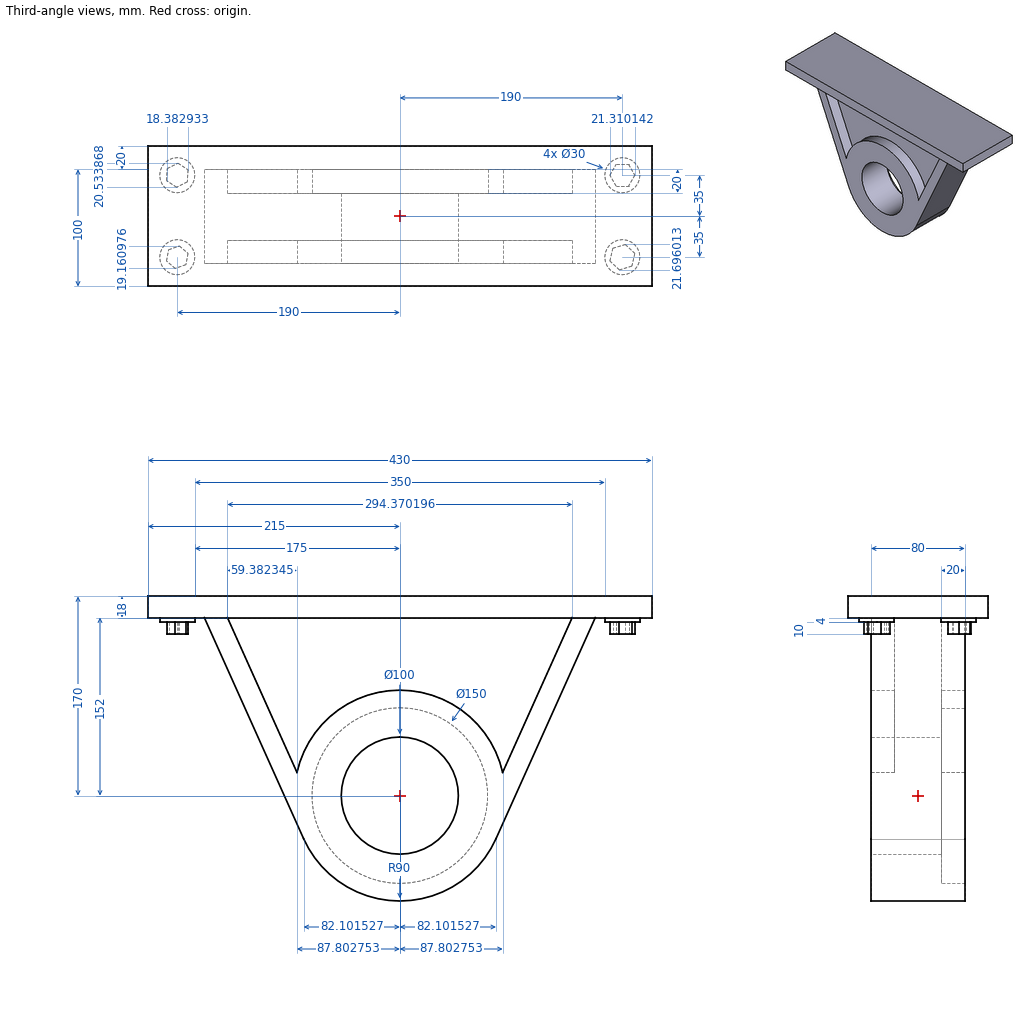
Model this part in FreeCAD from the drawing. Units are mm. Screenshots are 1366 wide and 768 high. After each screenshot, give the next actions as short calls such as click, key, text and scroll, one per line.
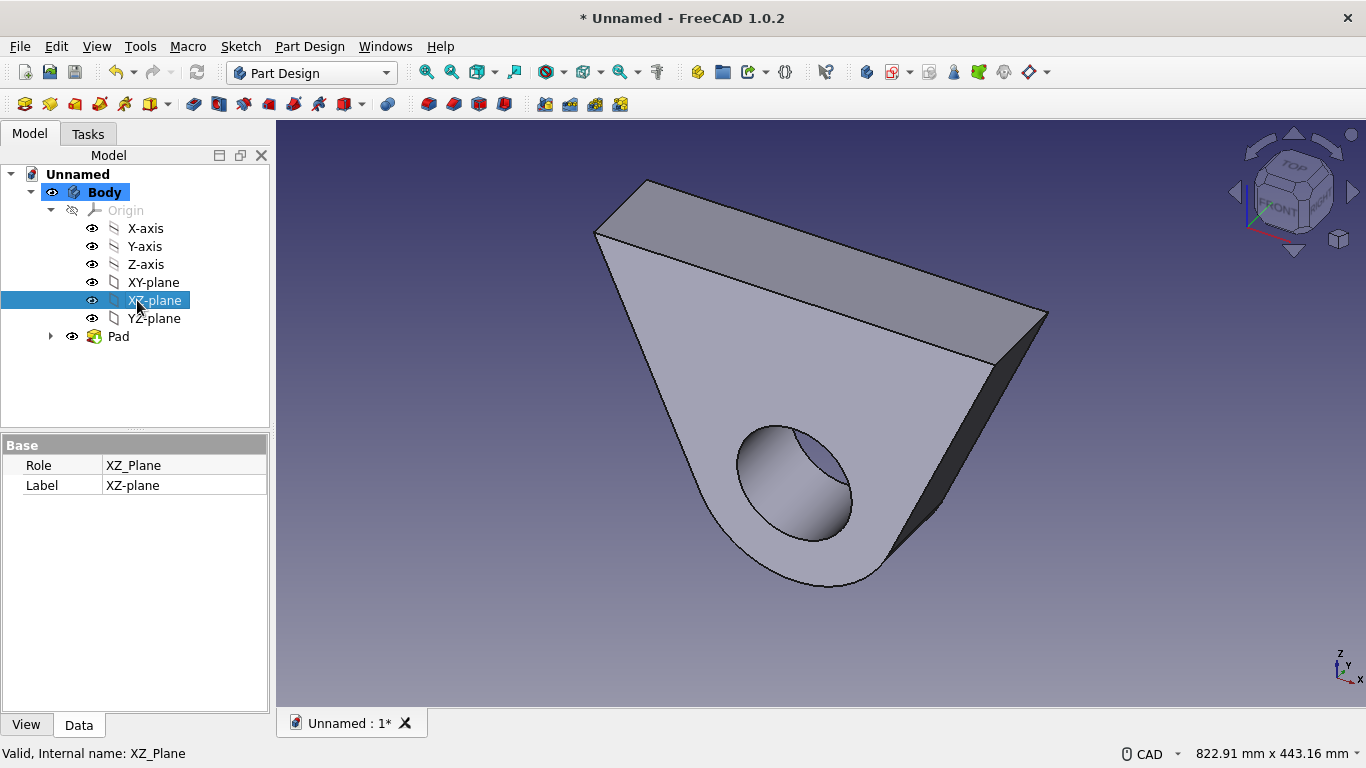
click(1028, 72)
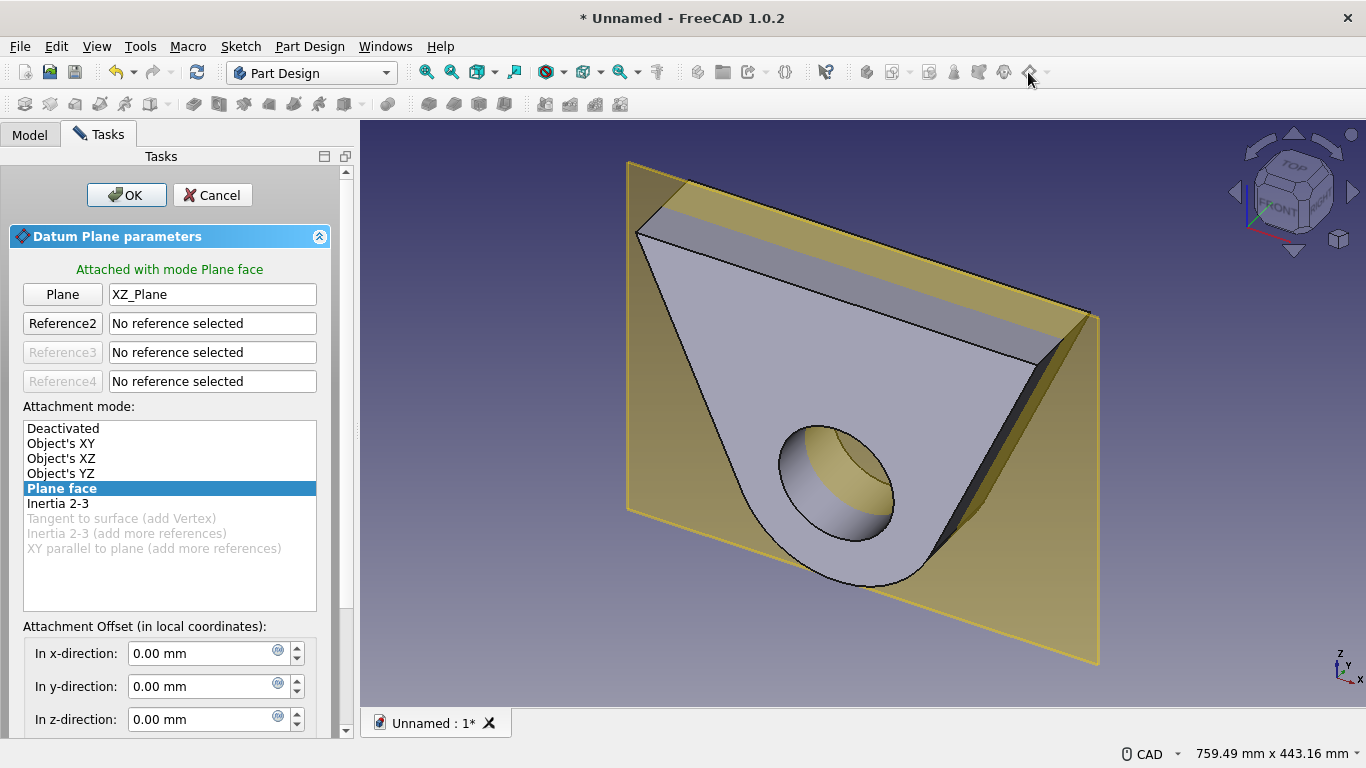
triple_click(210, 720)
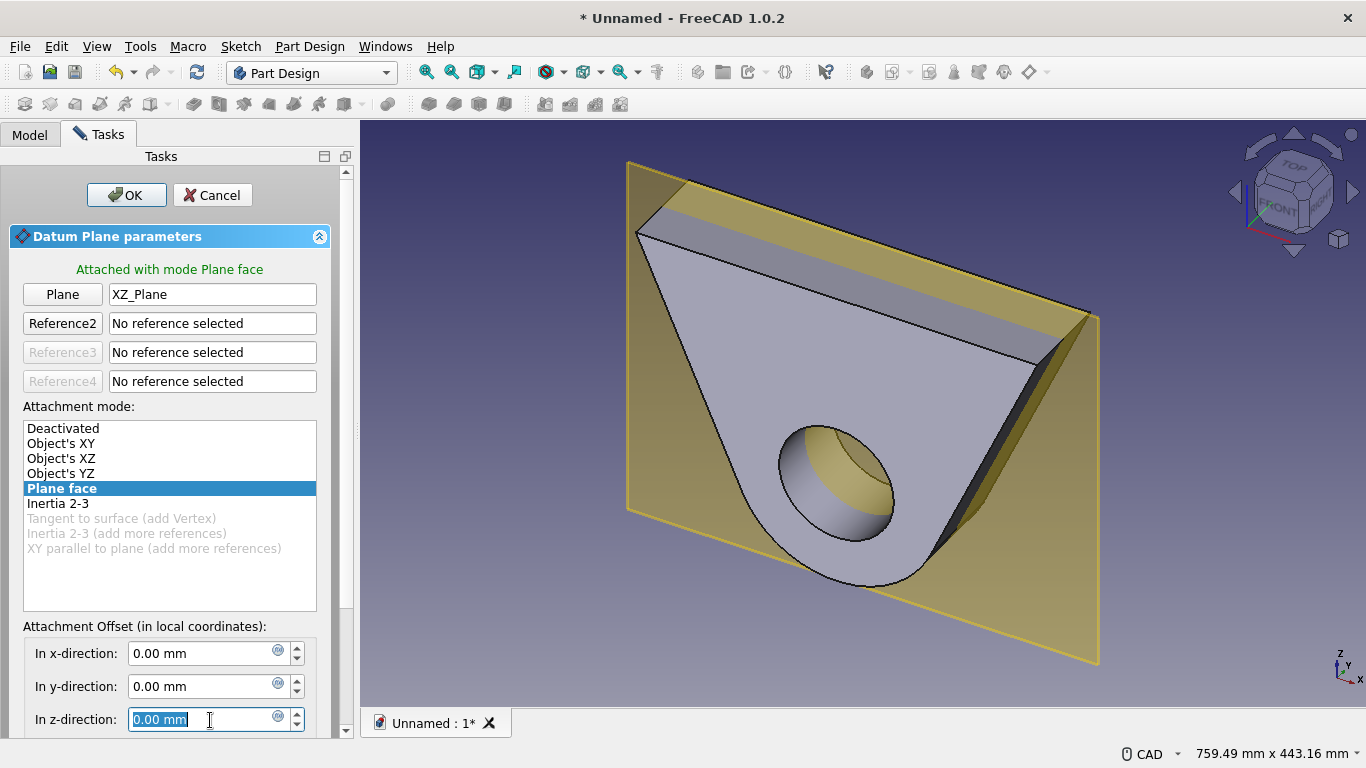
text(-20)
key(Tab)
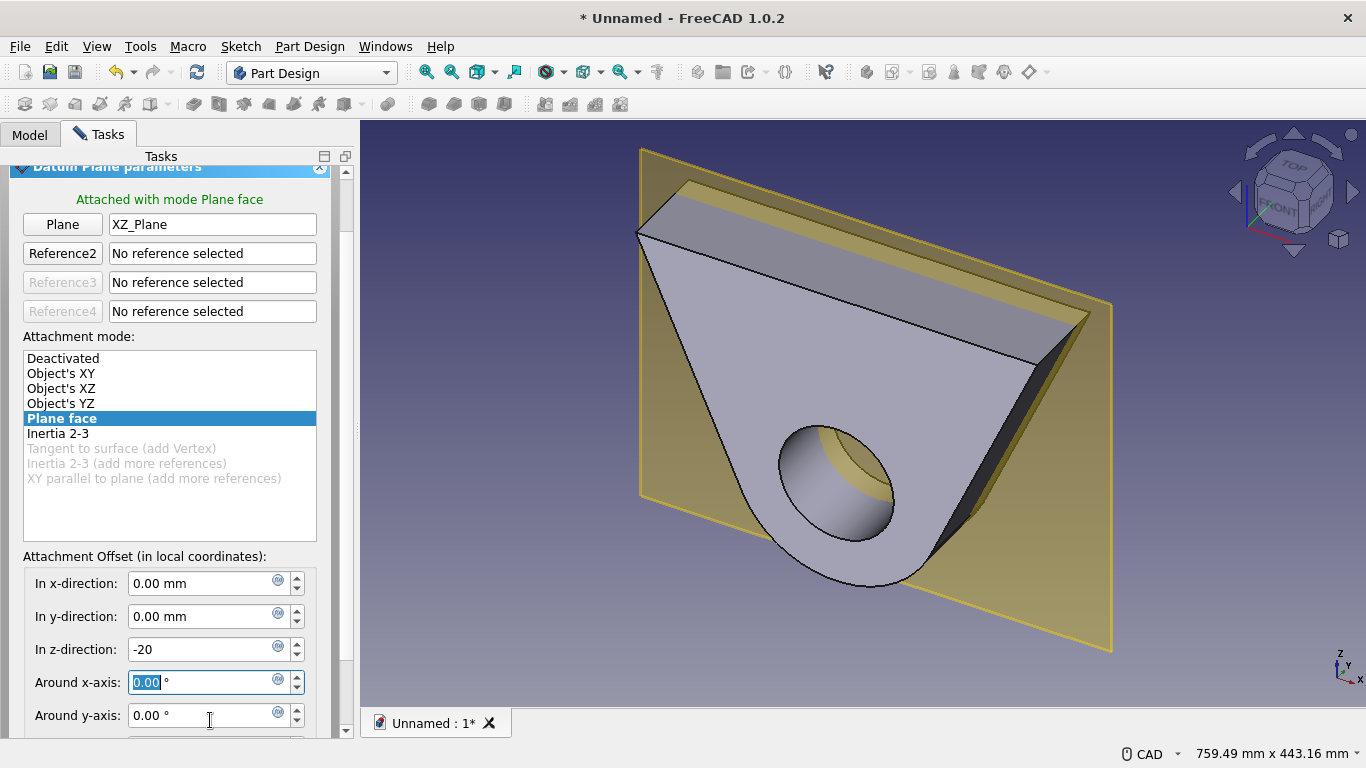
scroll(346, 452, up, 2)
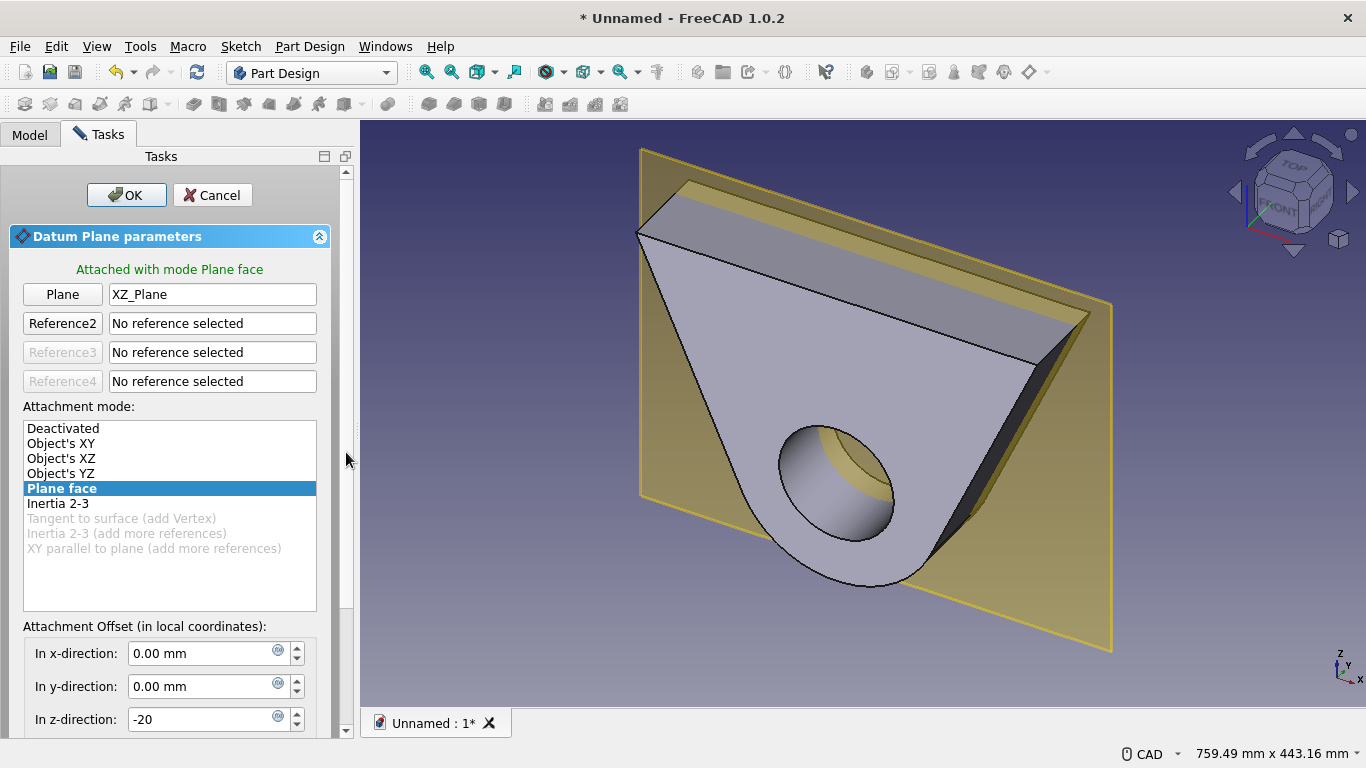
click(127, 195)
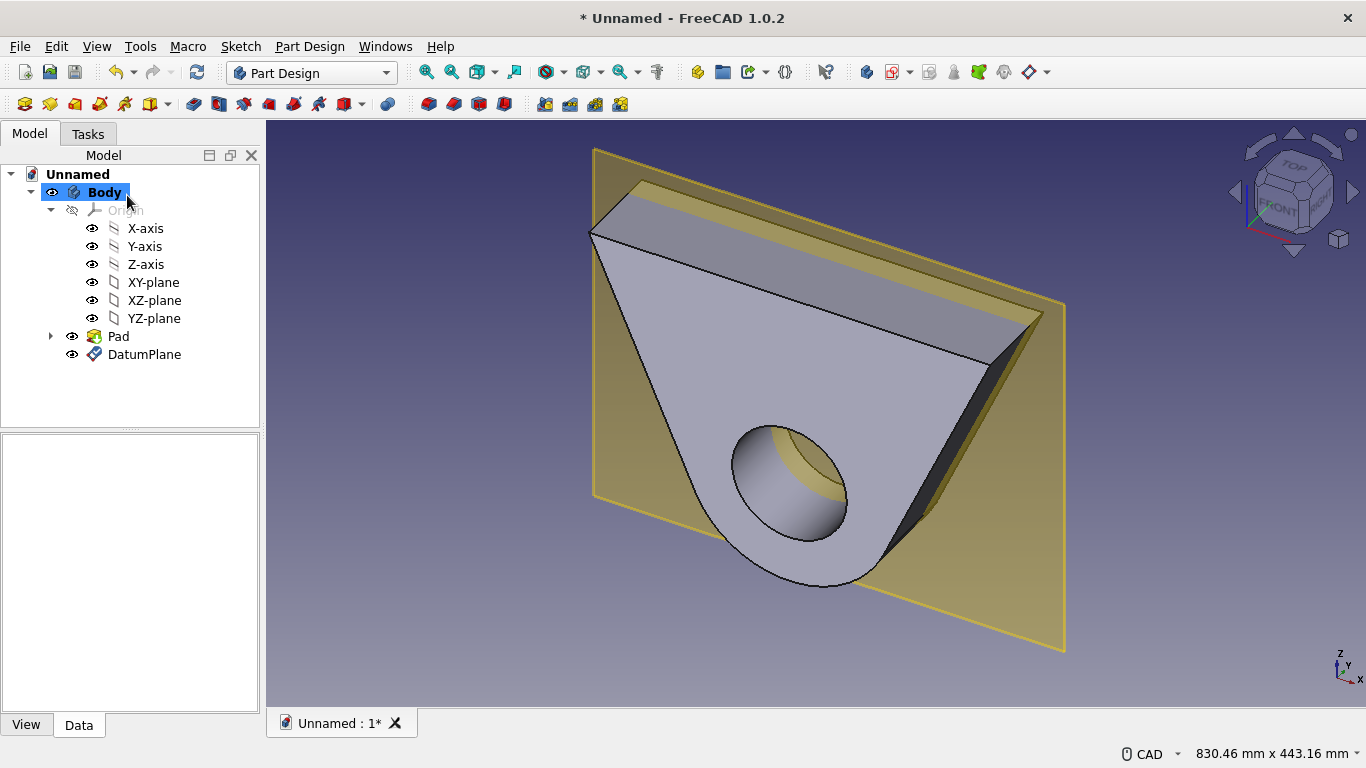
click(117, 354)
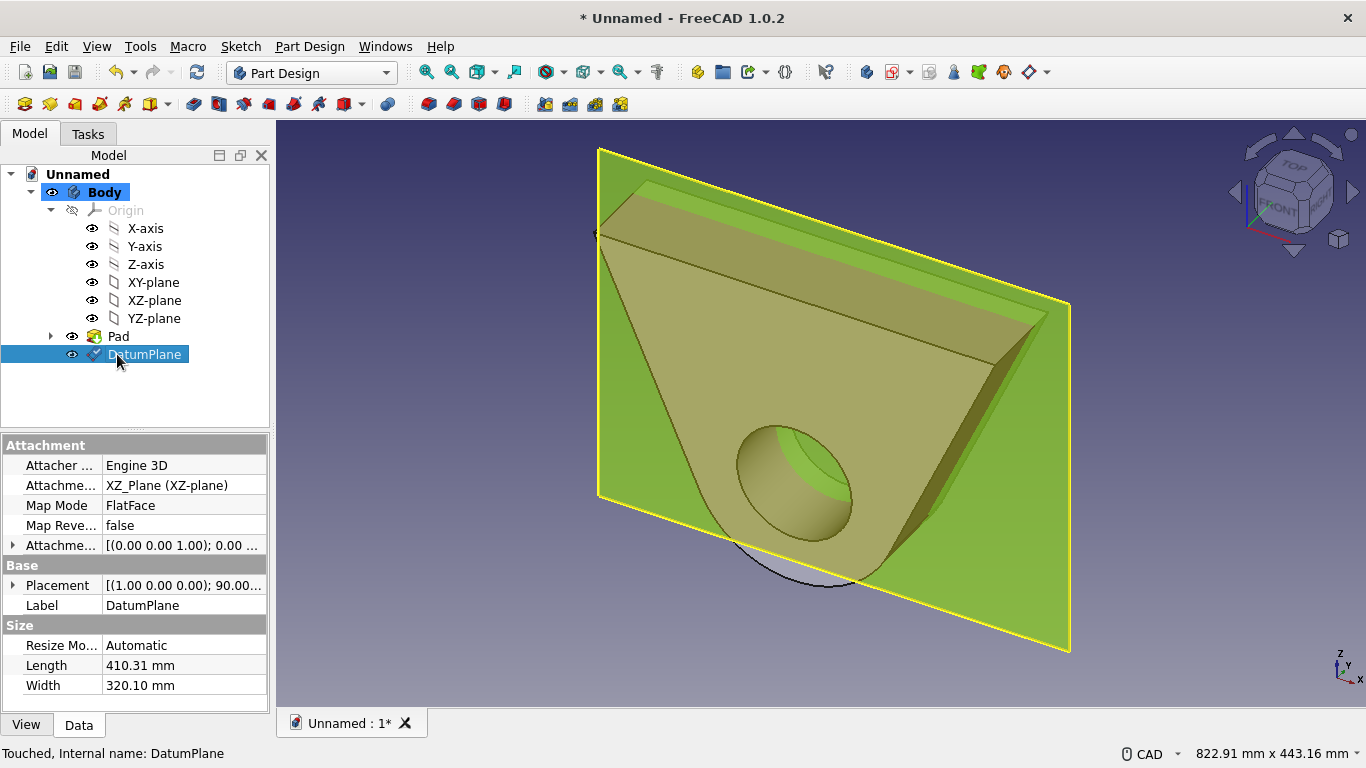
click(892, 72)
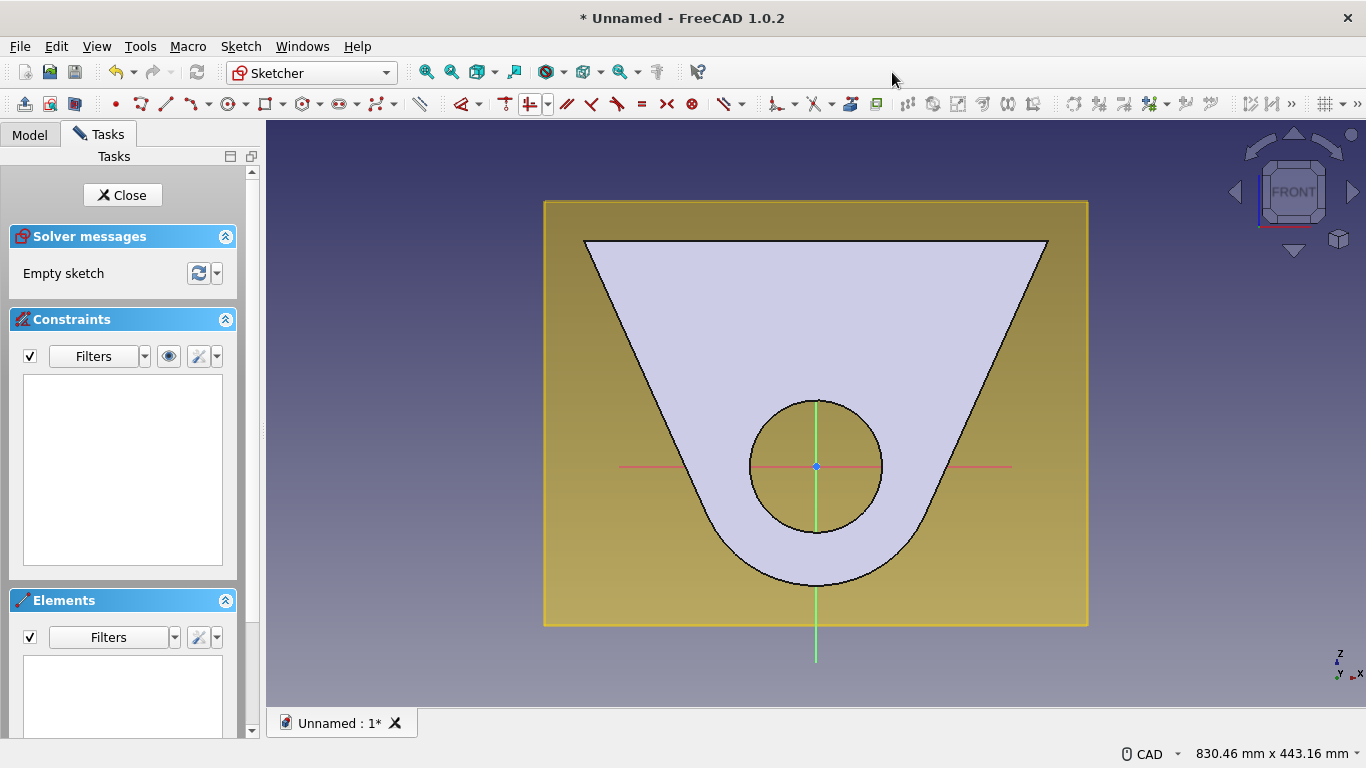
click(75, 104)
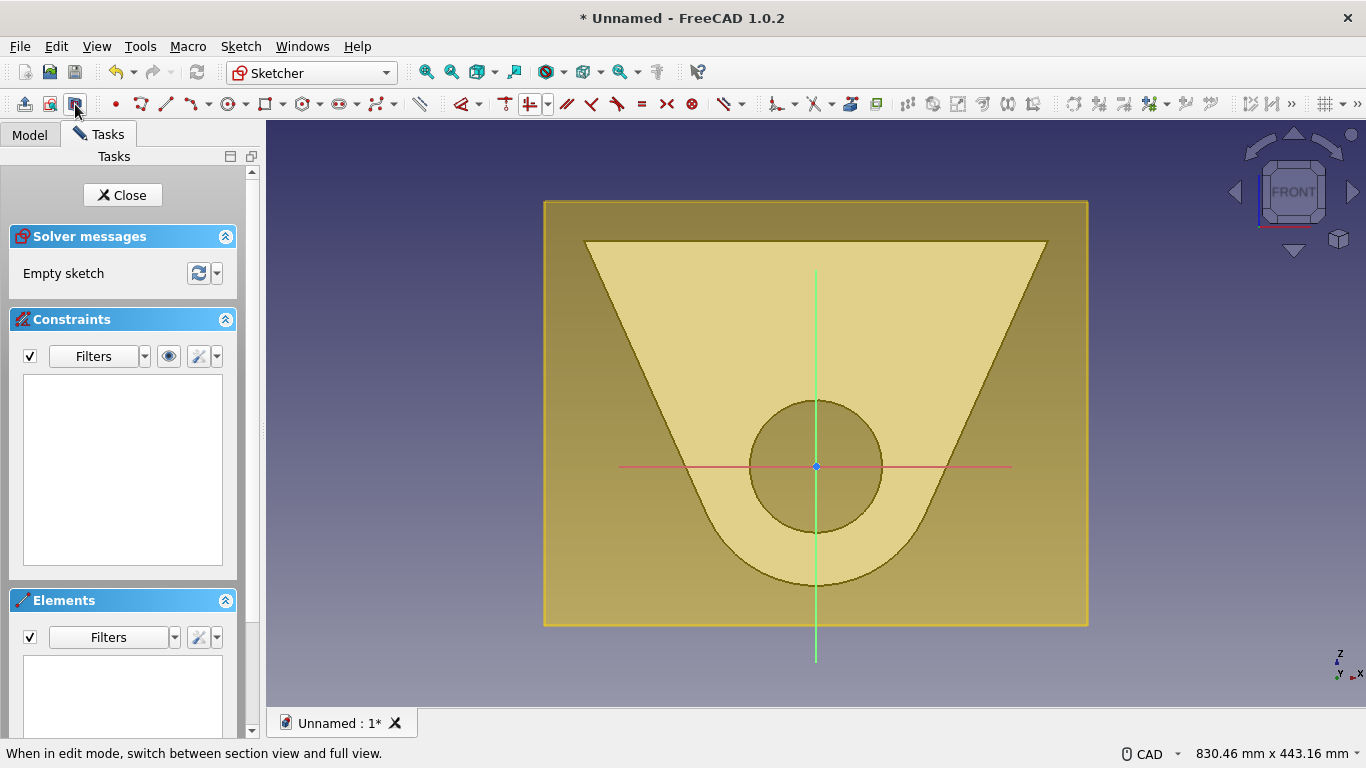
scroll(899, 531, up, 3)